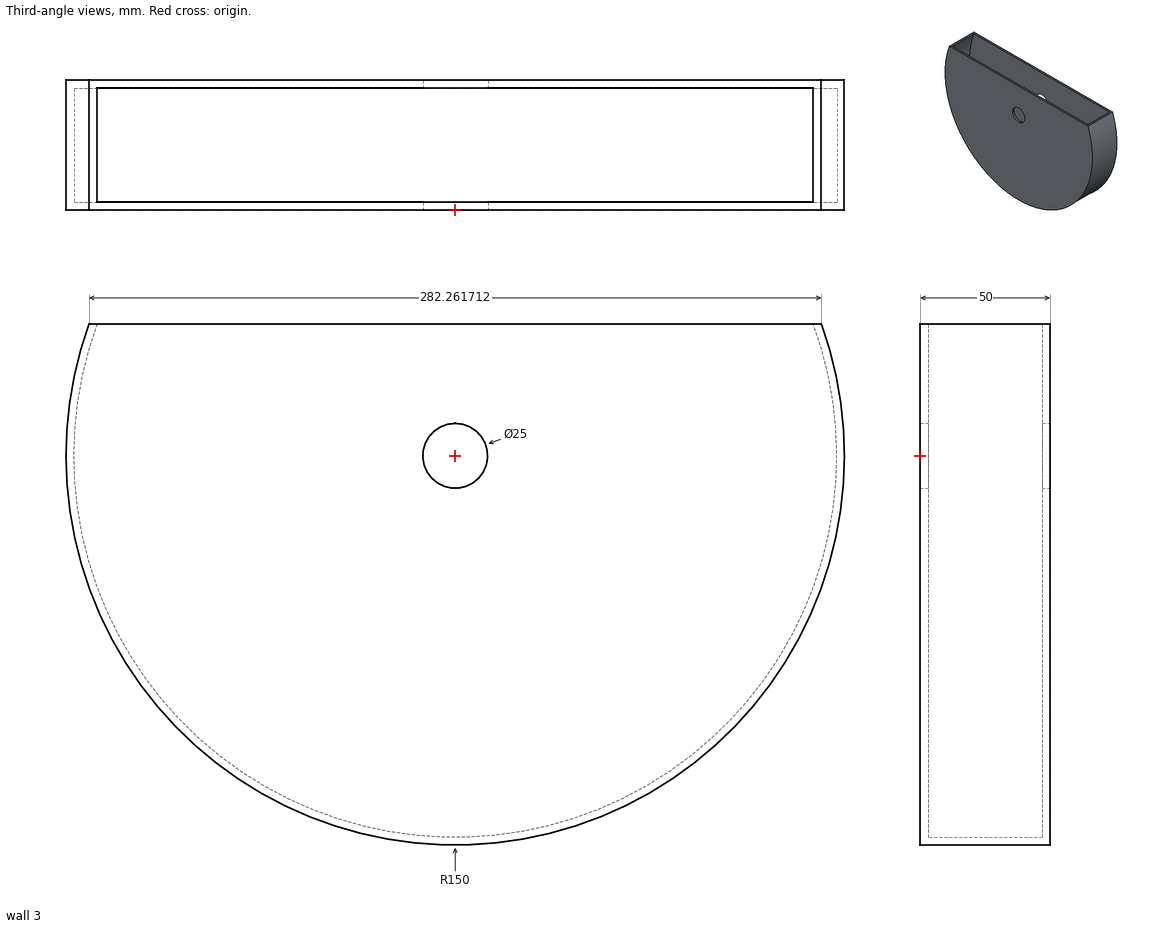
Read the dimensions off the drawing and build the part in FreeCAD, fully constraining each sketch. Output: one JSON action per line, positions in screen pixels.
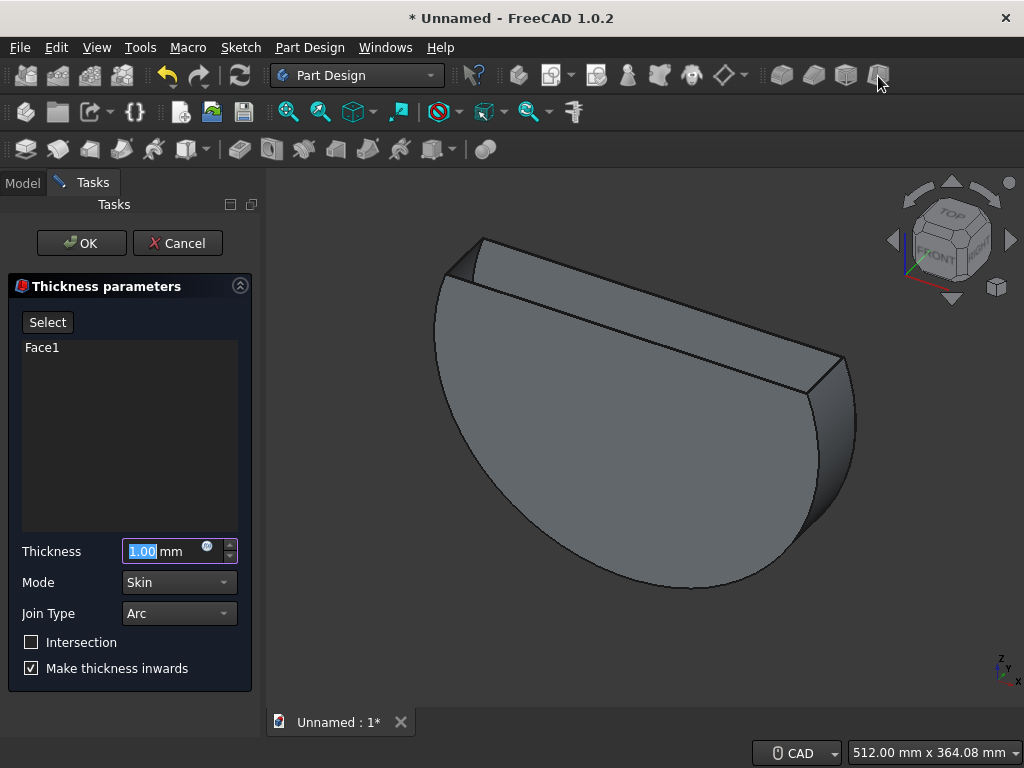
{"action": "type", "text": "3"}
{"action": "key", "text": "Tab"}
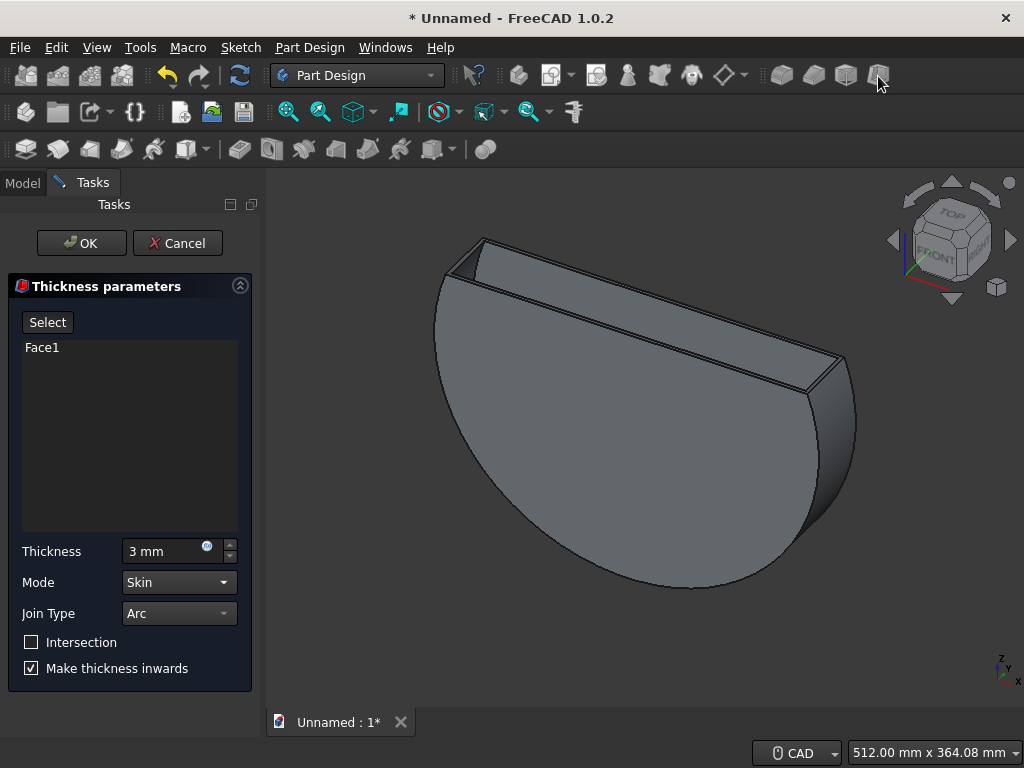
{"action": "left_click", "coordinate": [82, 243]}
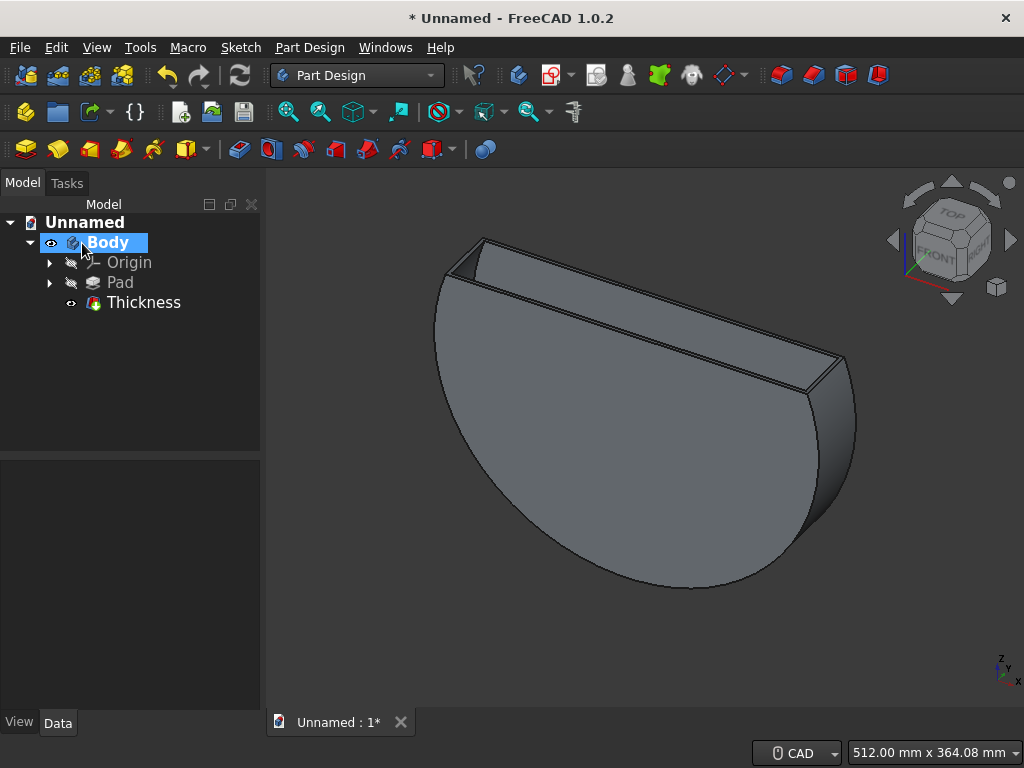
{"action": "key", "text": "4"}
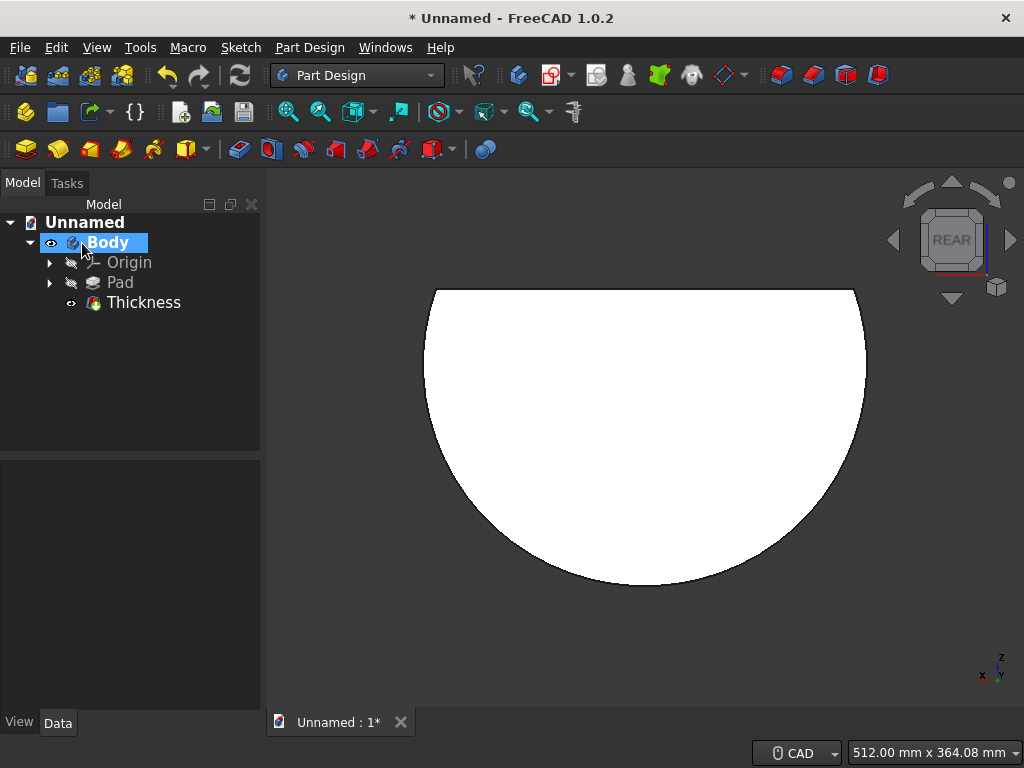
{"action": "left_click", "coordinate": [645, 437]}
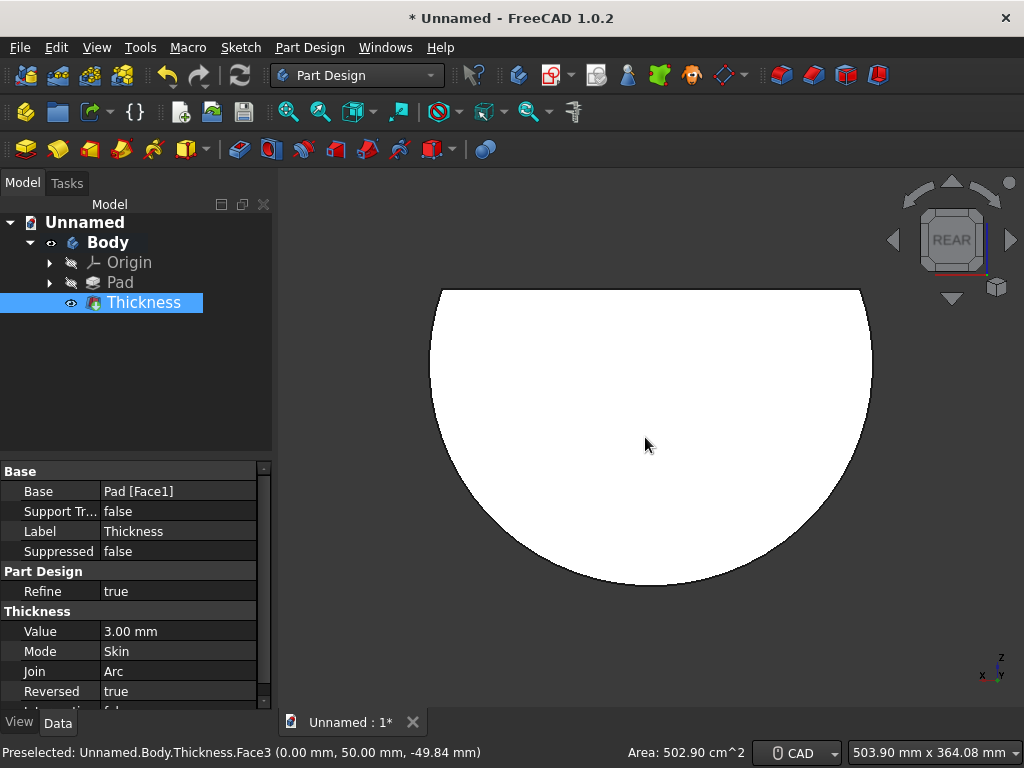
{"action": "left_click", "coordinate": [552, 76]}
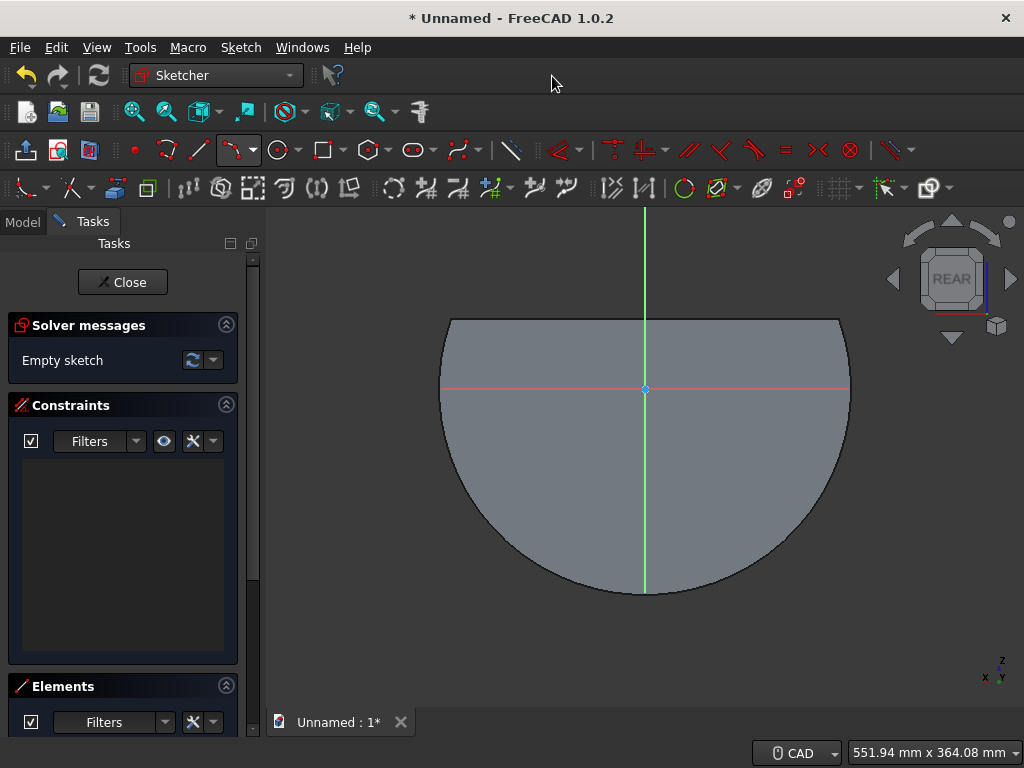
{"action": "scroll", "coordinate": [654, 381], "scroll_direction": "up", "scroll_amount": 11}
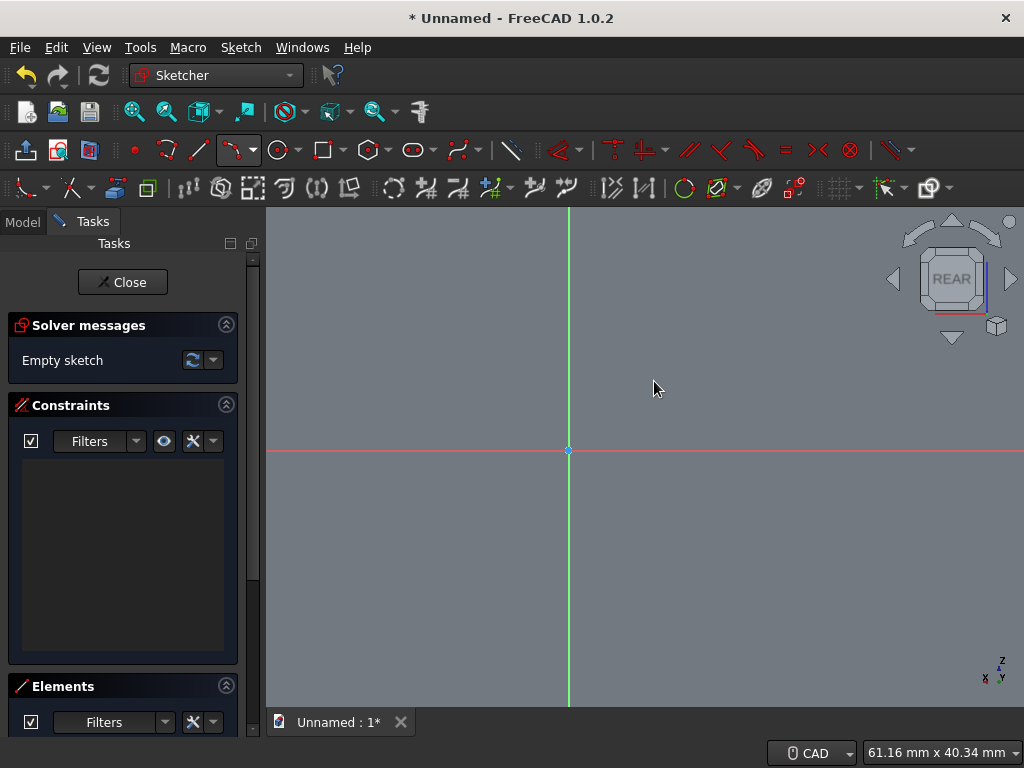
{"action": "left_click", "coordinate": [278, 150]}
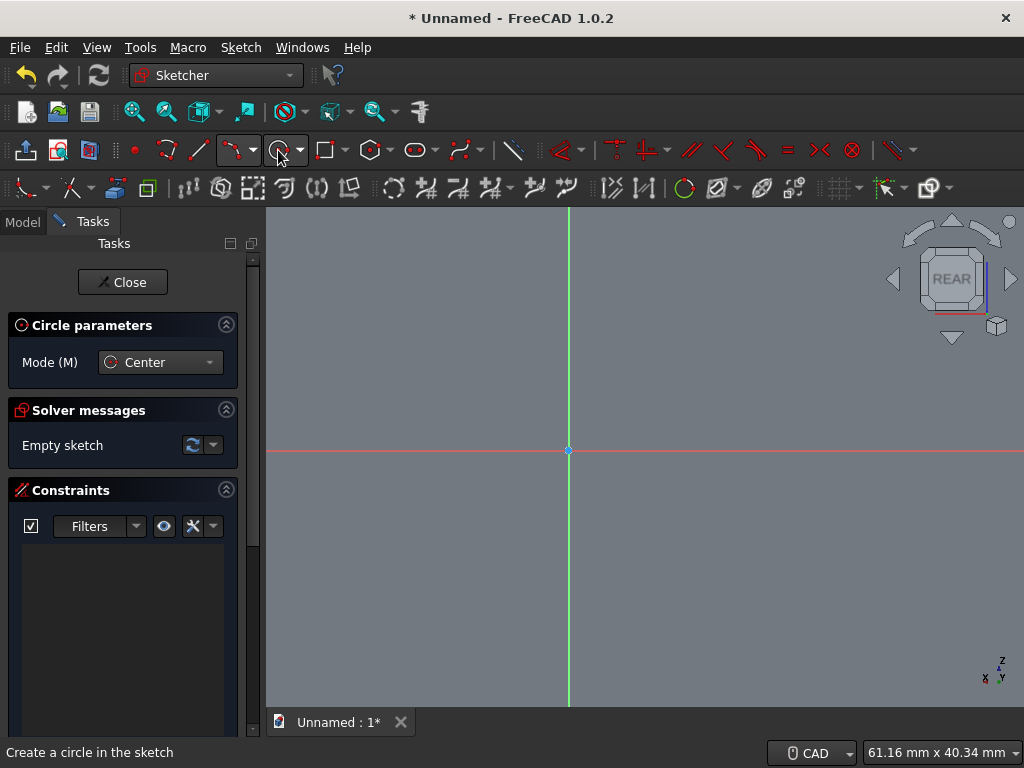
{"action": "left_click", "coordinate": [569, 451]}
{"action": "left_click", "coordinate": [678, 341]}
{"action": "key", "text": "Escape"}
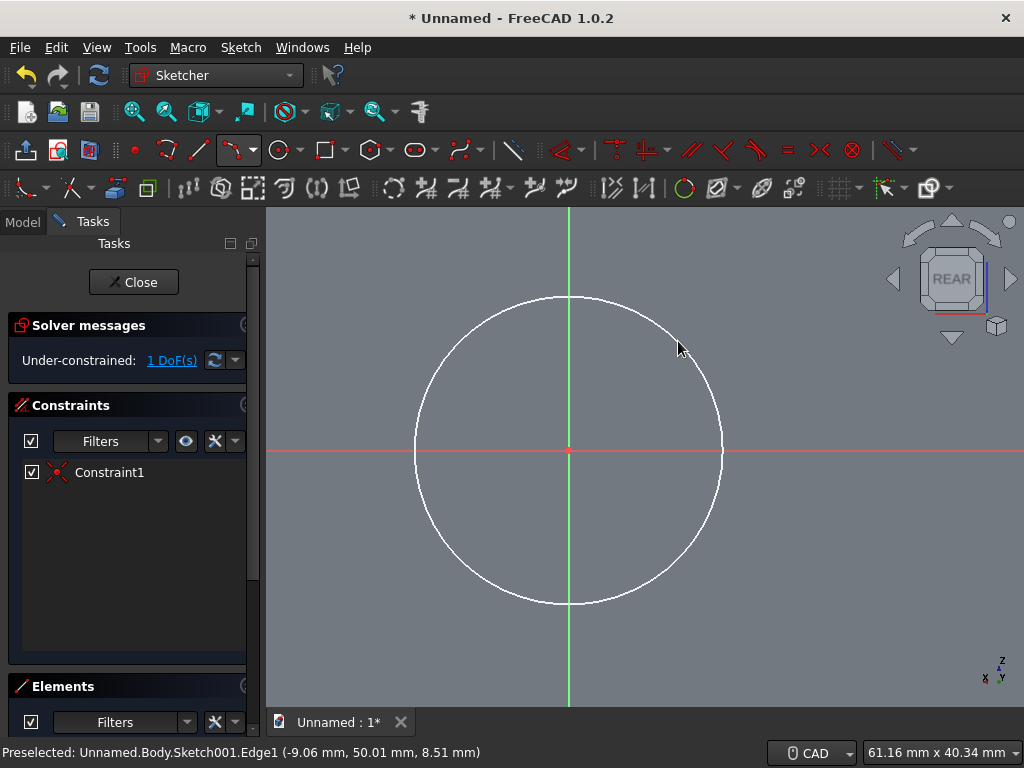
{"action": "key", "text": "d"}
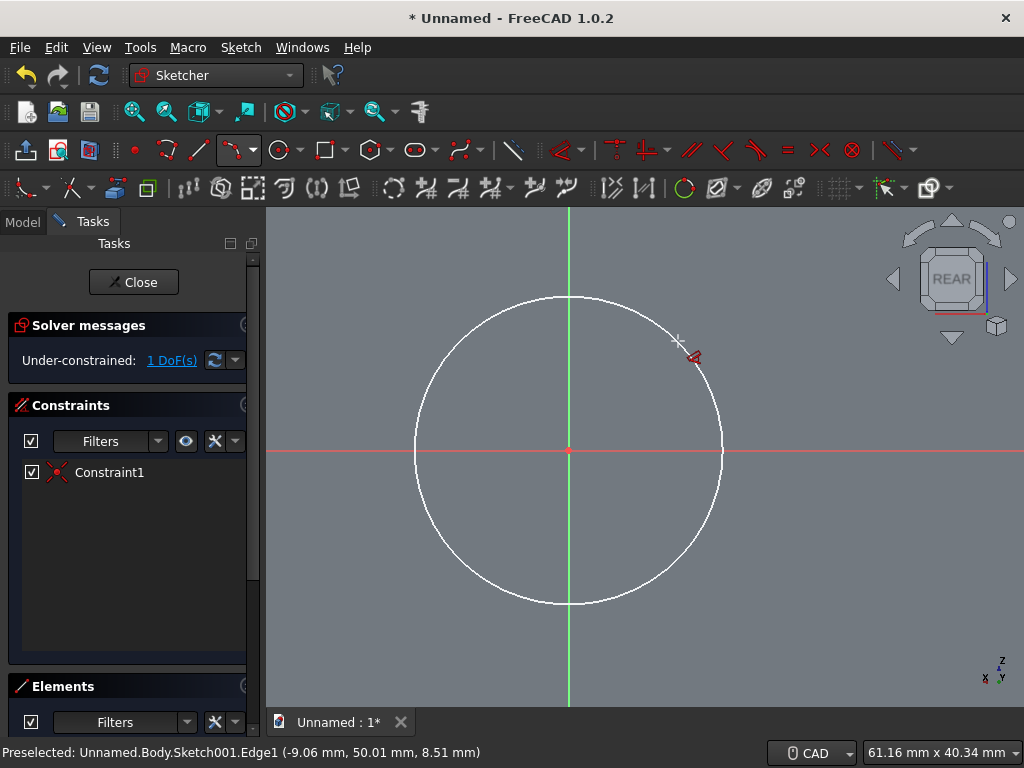
{"action": "left_click", "coordinate": [677, 341]}
{"action": "left_click", "coordinate": [700, 318]}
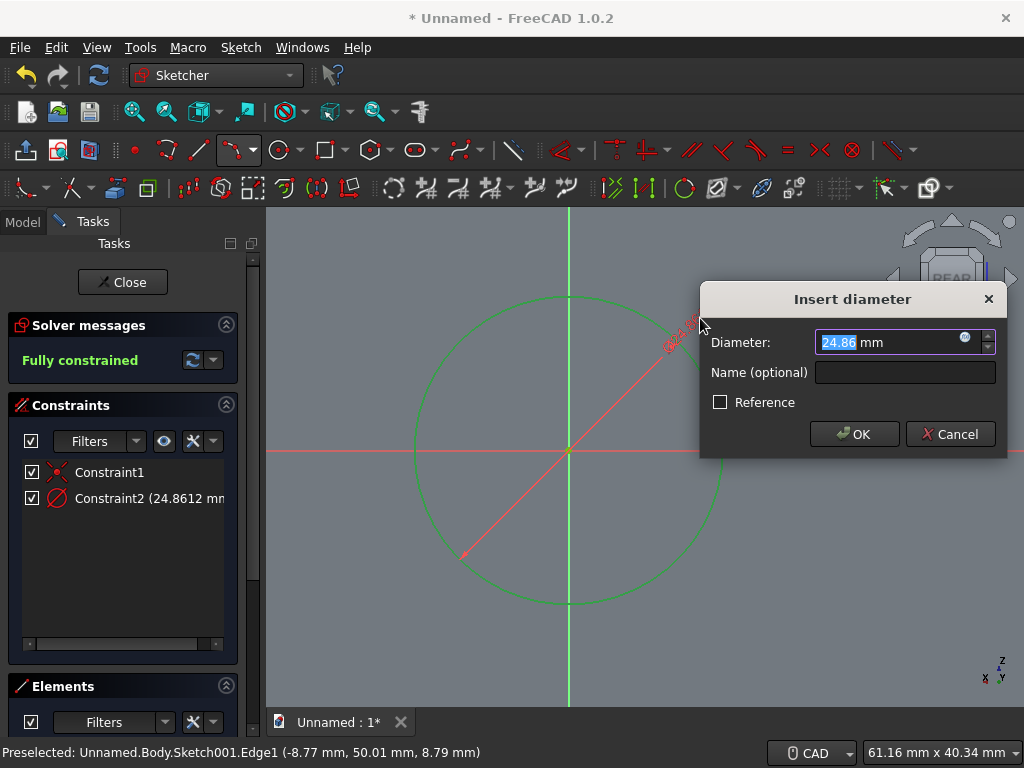
{"action": "type", "text": "25"}
{"action": "key", "text": "Return"}
{"action": "key", "text": "Escape"}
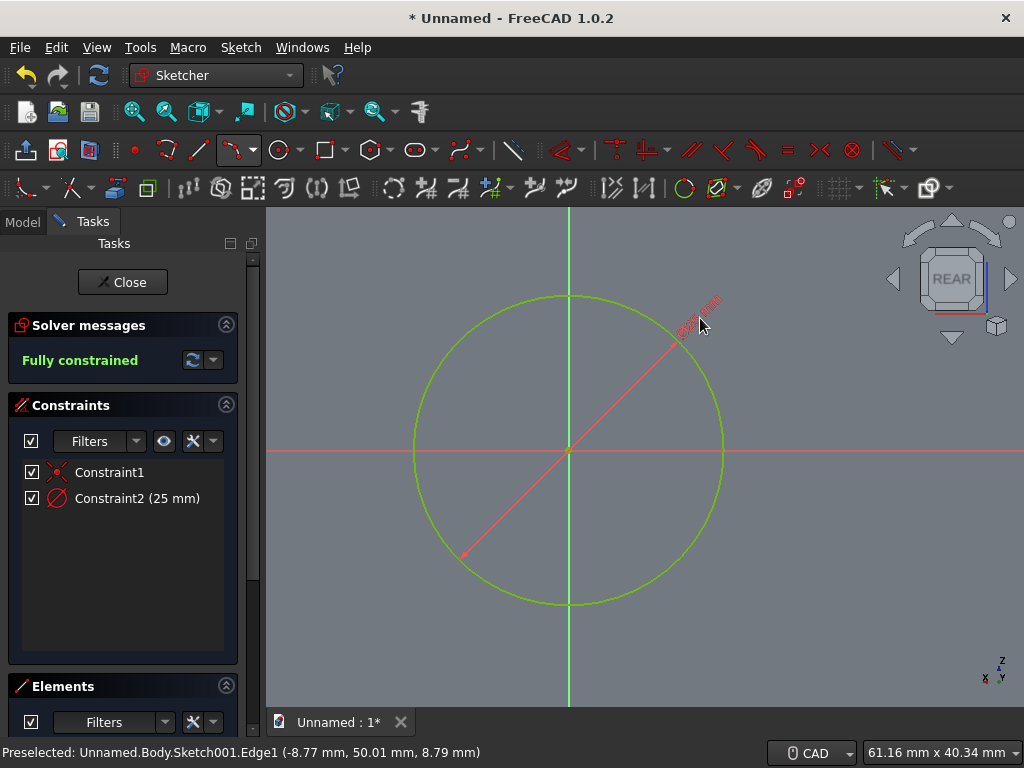
{"action": "left_click", "coordinate": [123, 282]}